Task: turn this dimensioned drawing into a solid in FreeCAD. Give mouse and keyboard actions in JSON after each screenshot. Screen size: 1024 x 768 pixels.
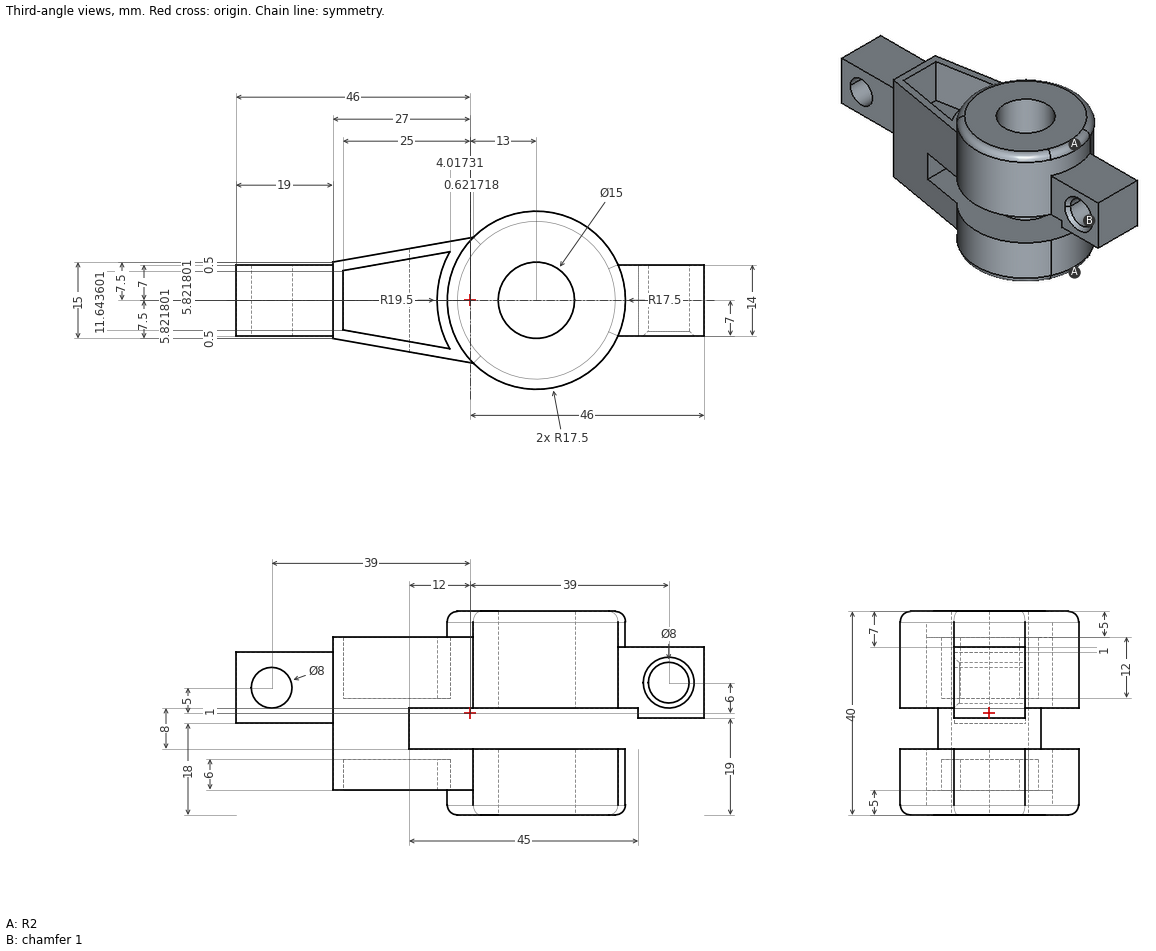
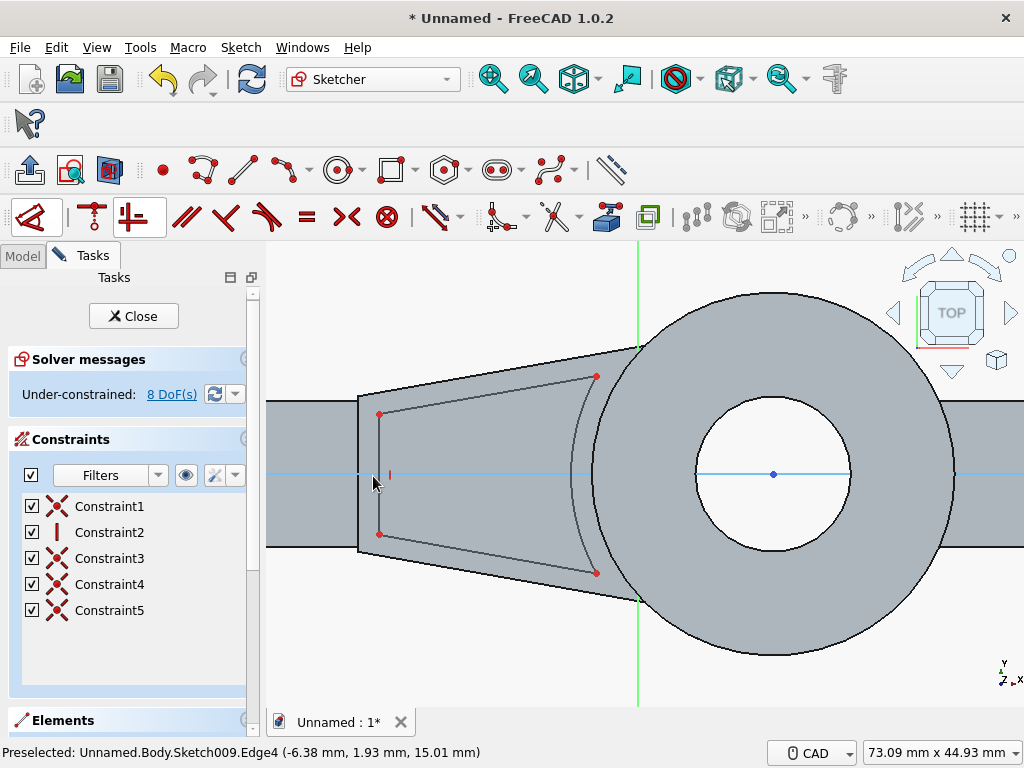
{"action": "left_click", "coordinate": [774, 475]}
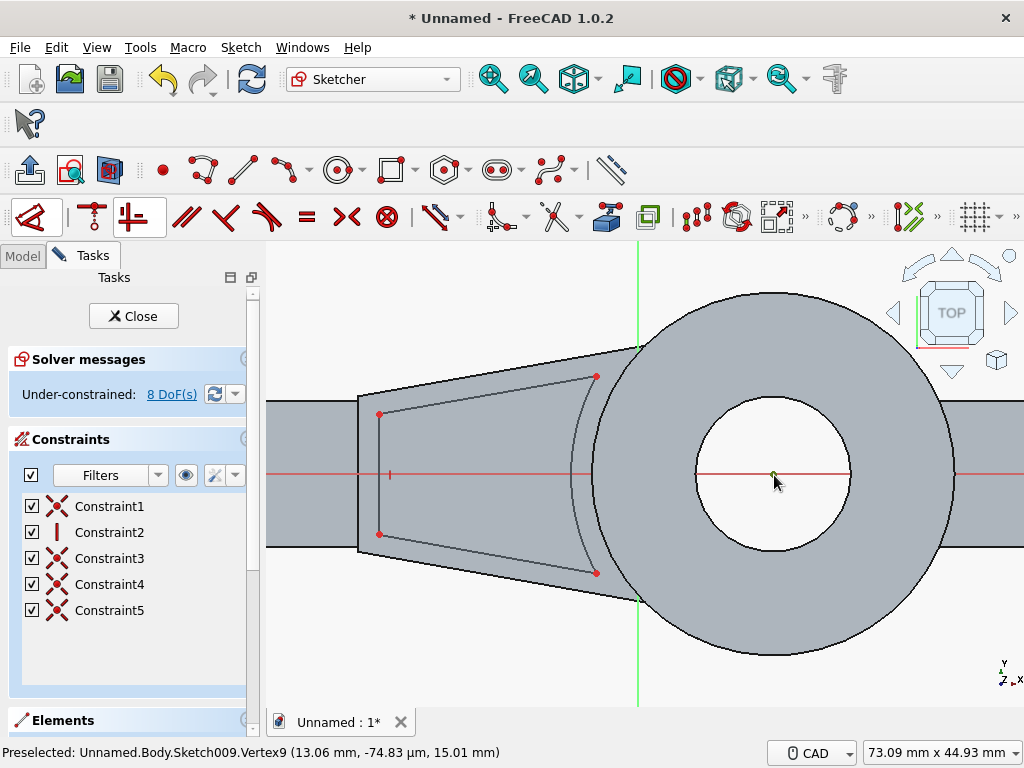
{"action": "left_click", "coordinate": [334, 474]}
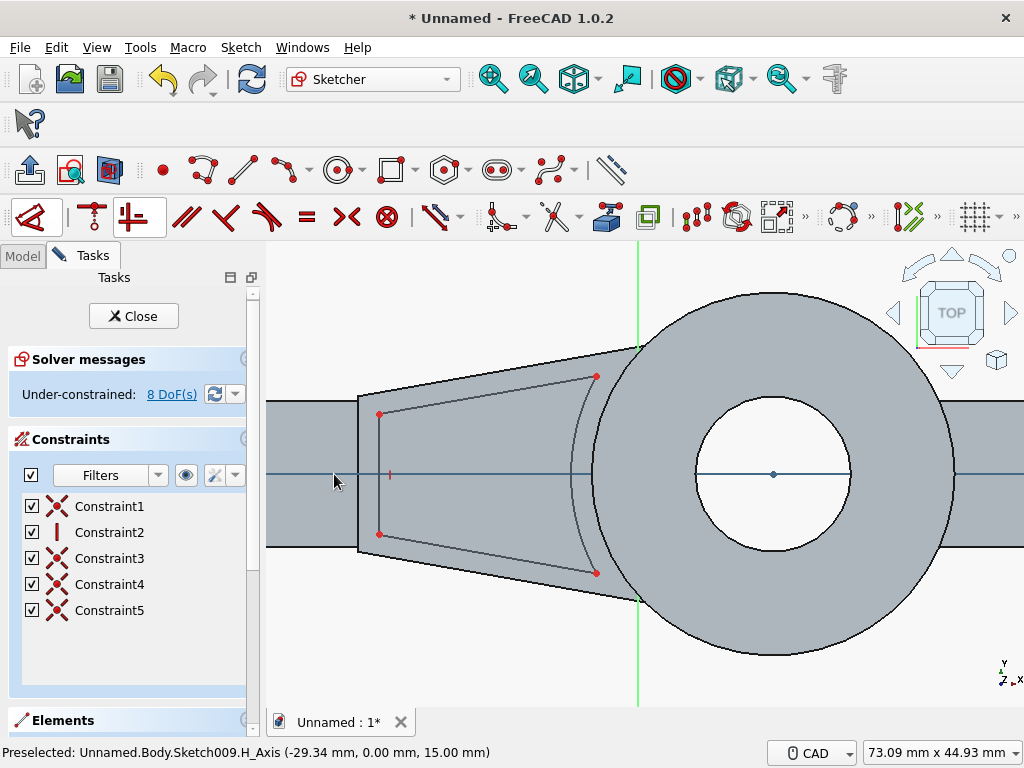
{"action": "left_click", "coordinate": [92, 218]}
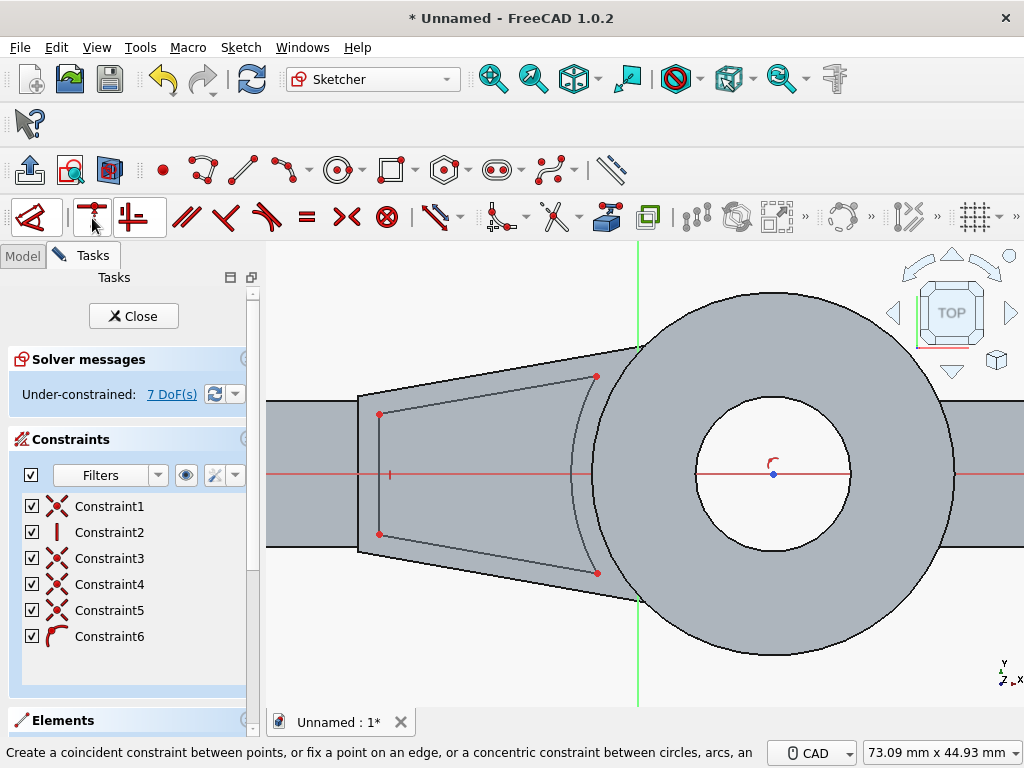
{"action": "left_click", "coordinate": [575, 434]}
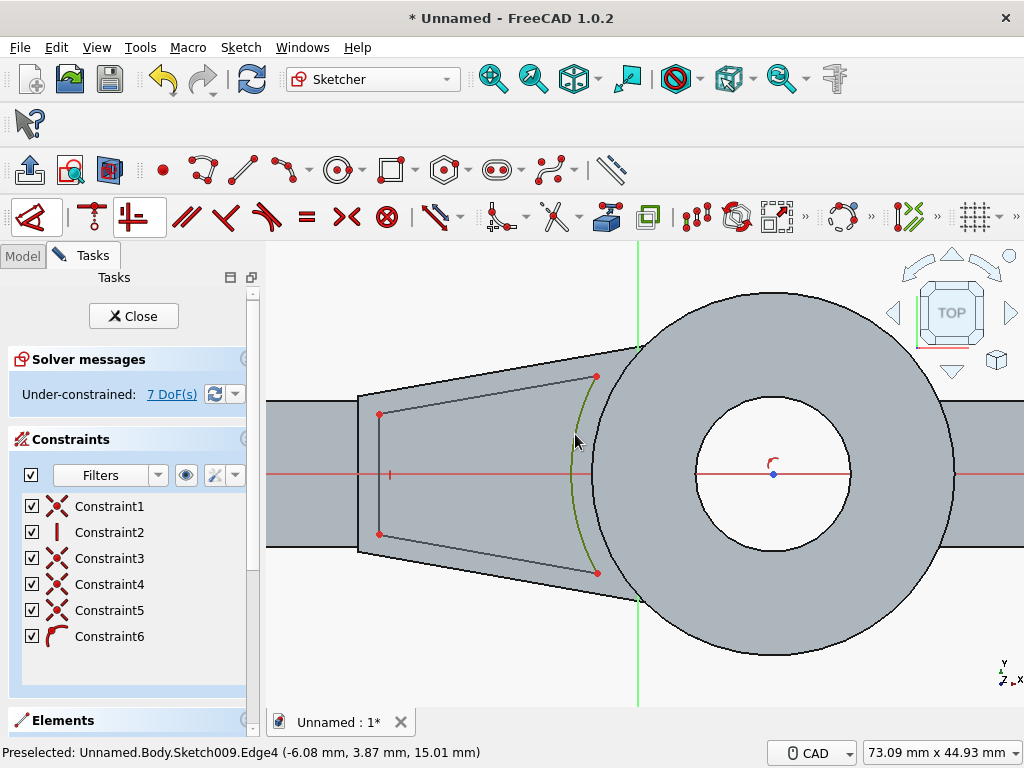
{"action": "left_click", "coordinate": [56, 218]}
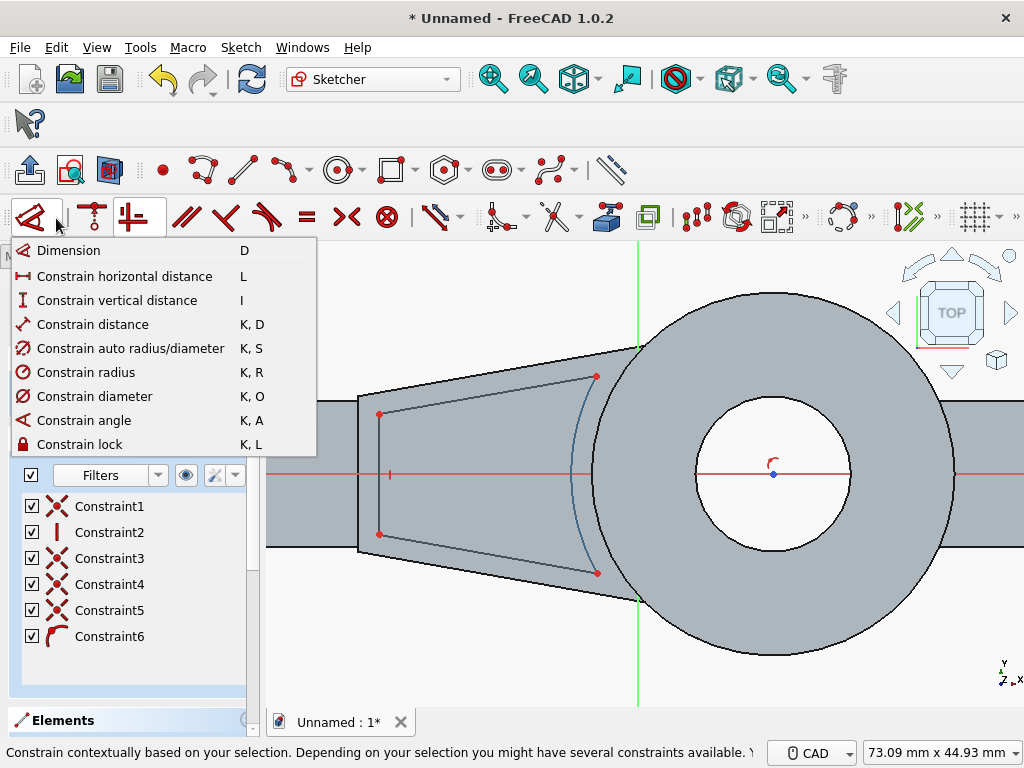
{"action": "left_click", "coordinate": [164, 372]}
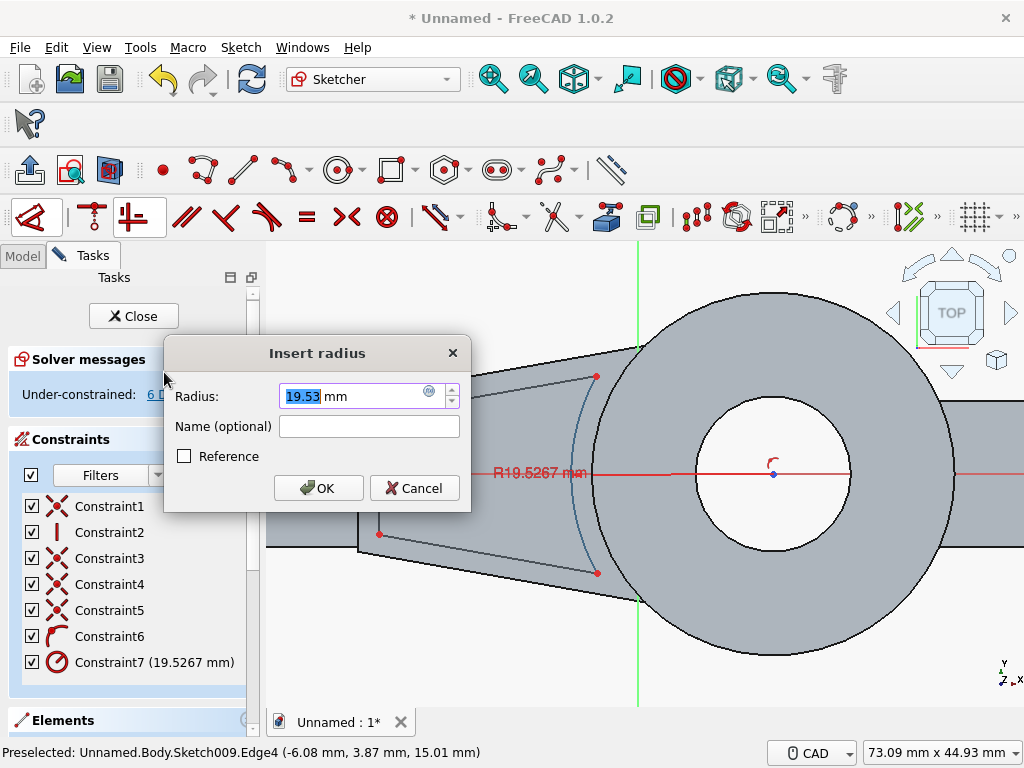
{"action": "type", "text": "19.5"}
{"action": "key", "text": "Return"}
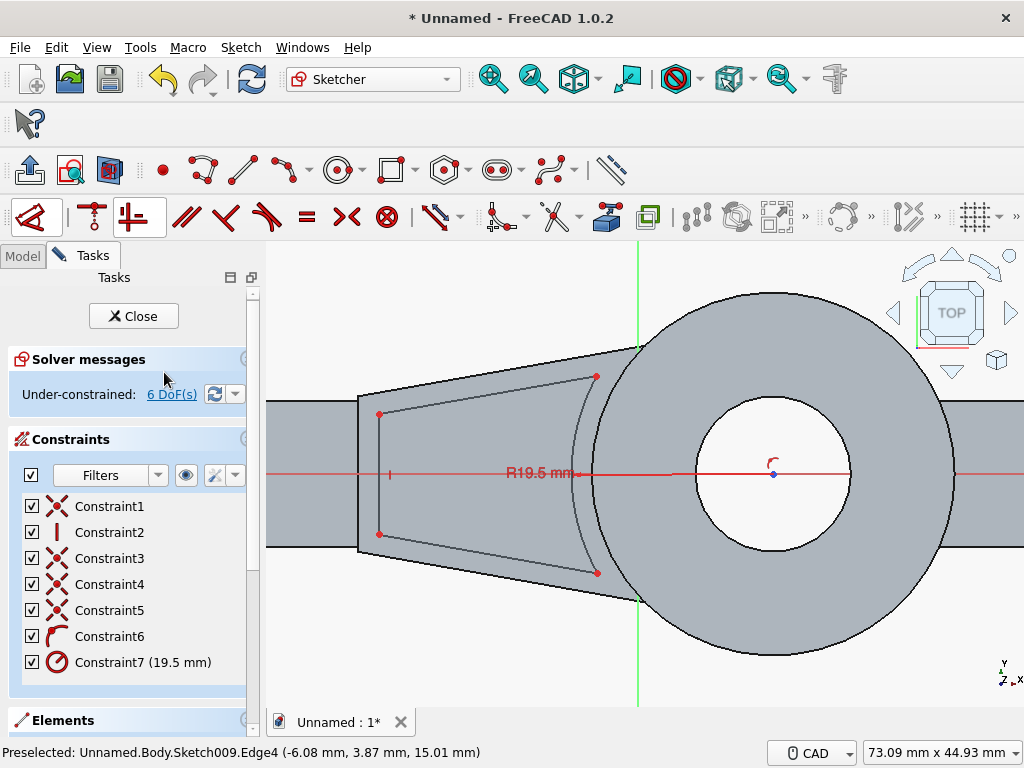
{"action": "left_click", "coordinate": [379, 414]}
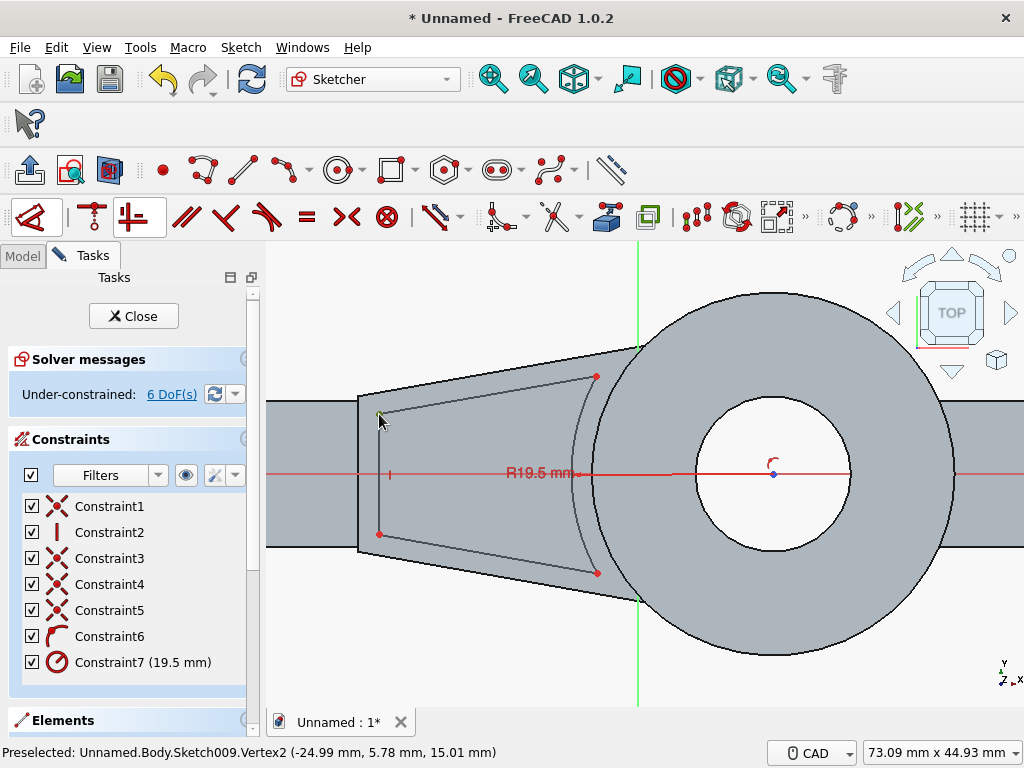
{"action": "left_click", "coordinate": [56, 218]}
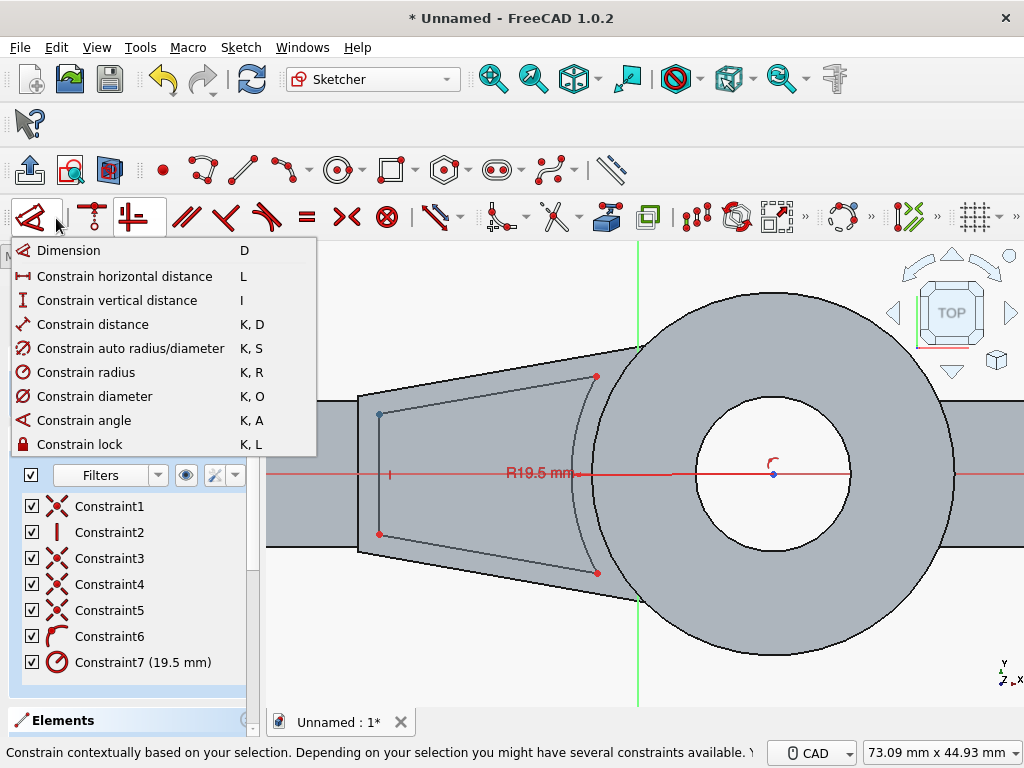
{"action": "left_click", "coordinate": [164, 276]}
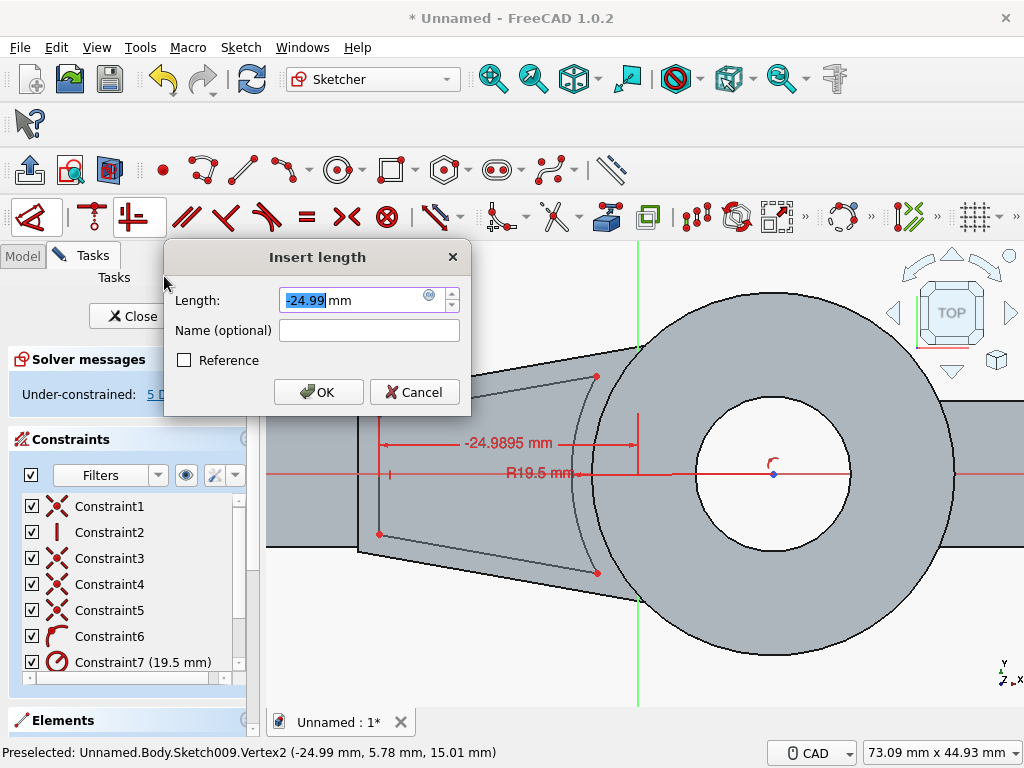
{"action": "type", "text": "-25"}
{"action": "key", "text": "Return"}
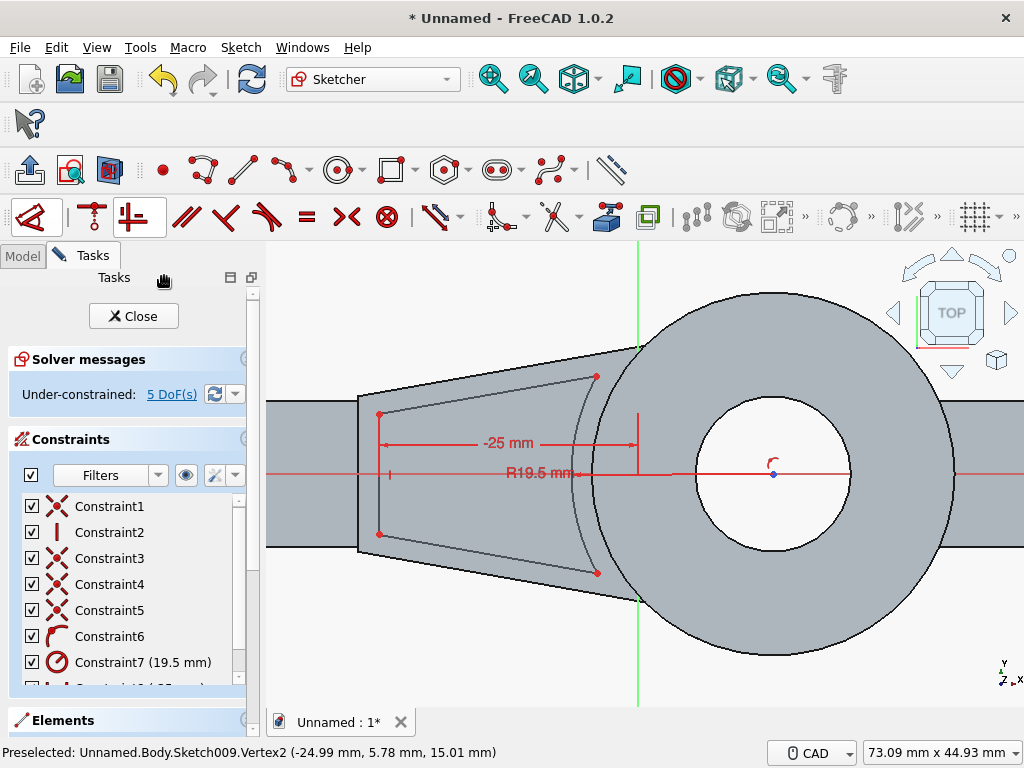
{"action": "left_click", "coordinate": [774, 474]}